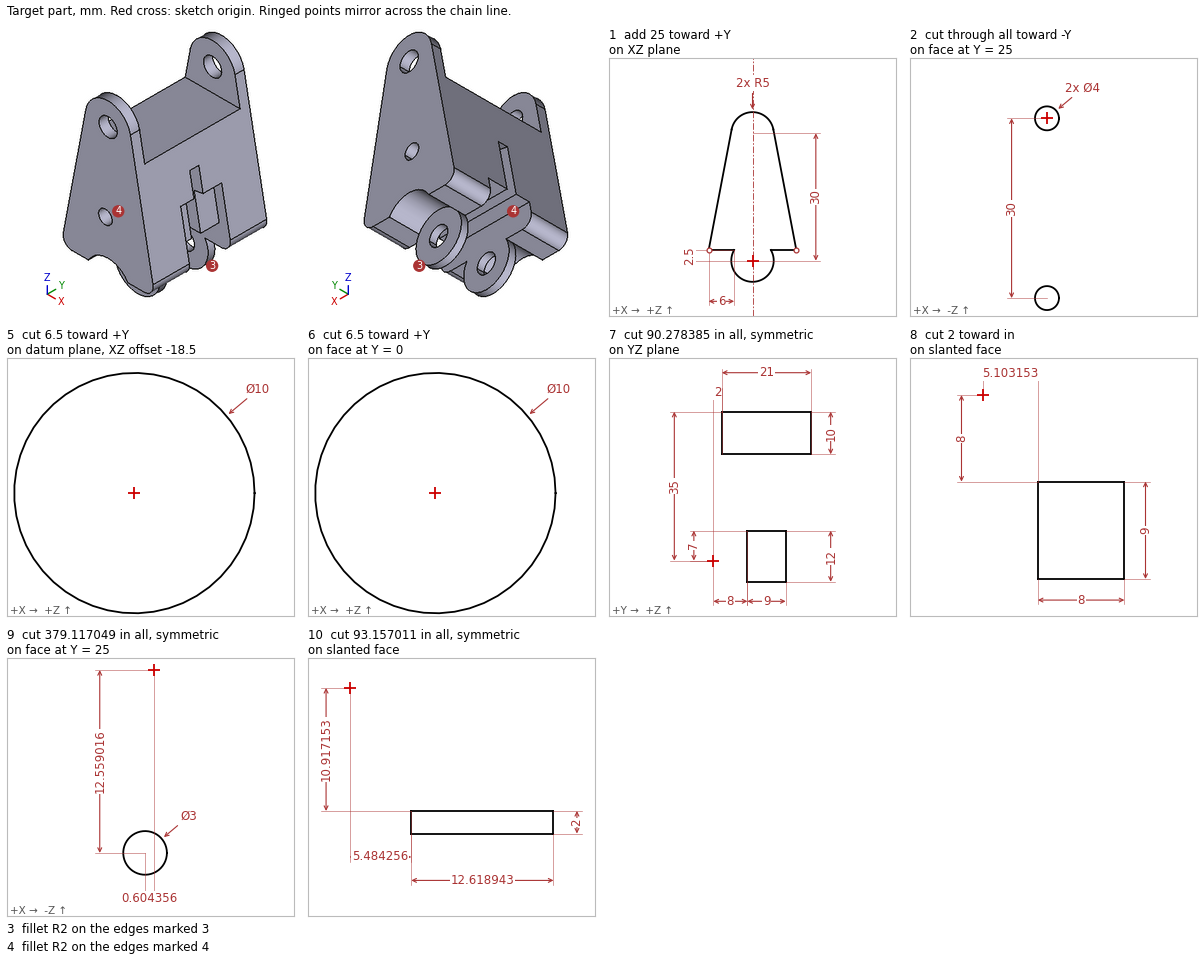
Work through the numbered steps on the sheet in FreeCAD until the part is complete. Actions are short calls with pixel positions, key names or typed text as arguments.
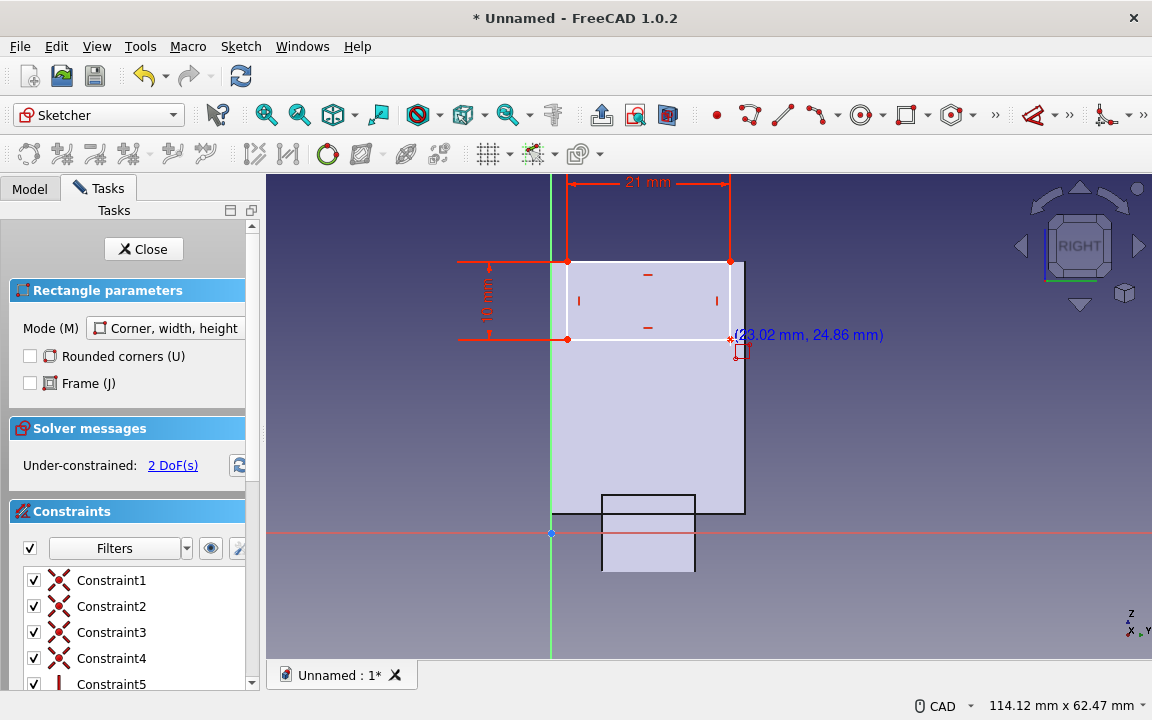
click(613, 479)
move(683, 572)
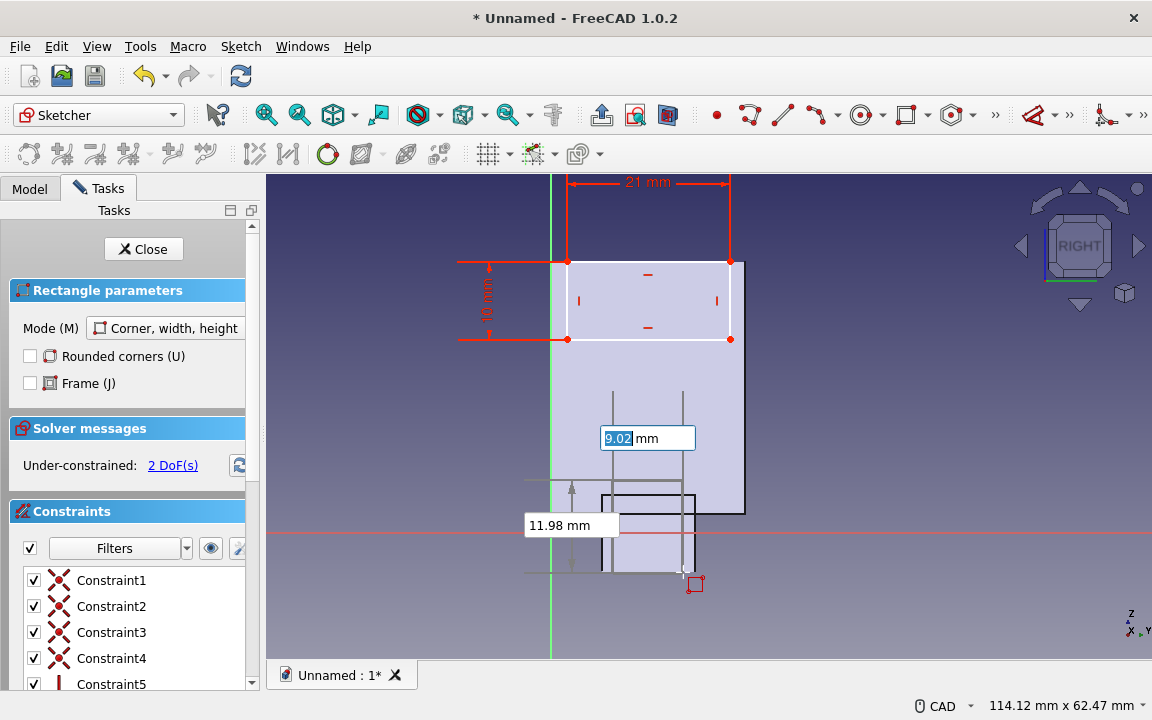
text(9)
key(Tab)
text(12)
key(Return)
key(Escape)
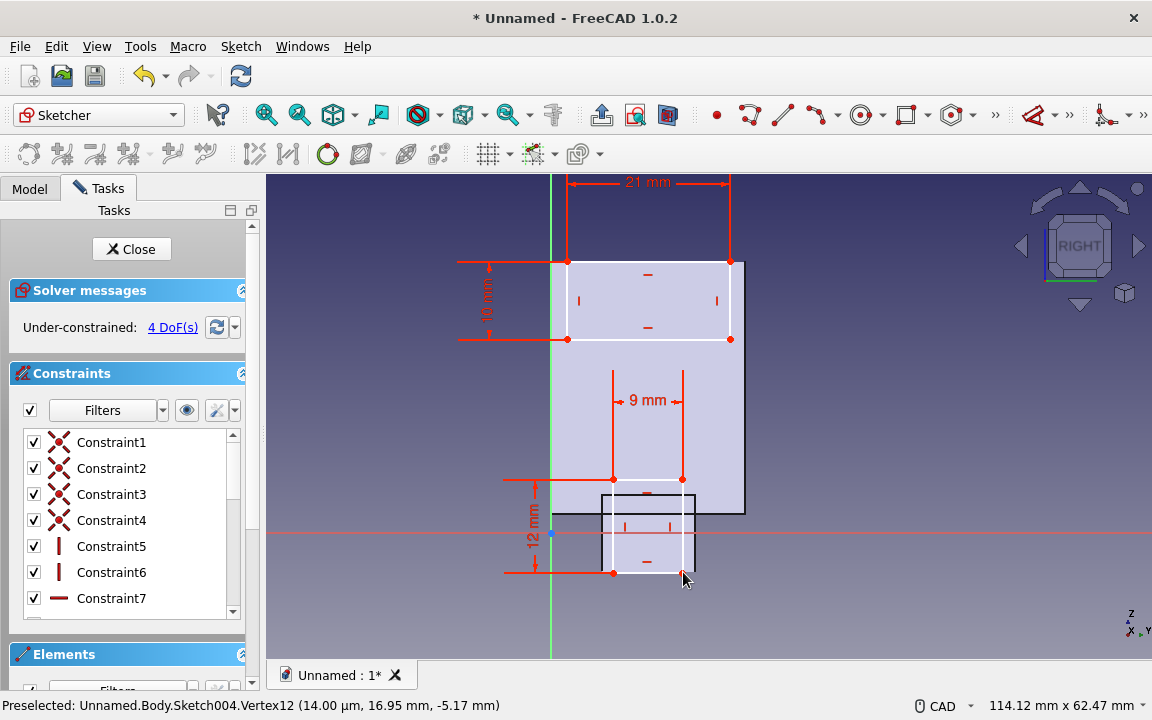
key(d)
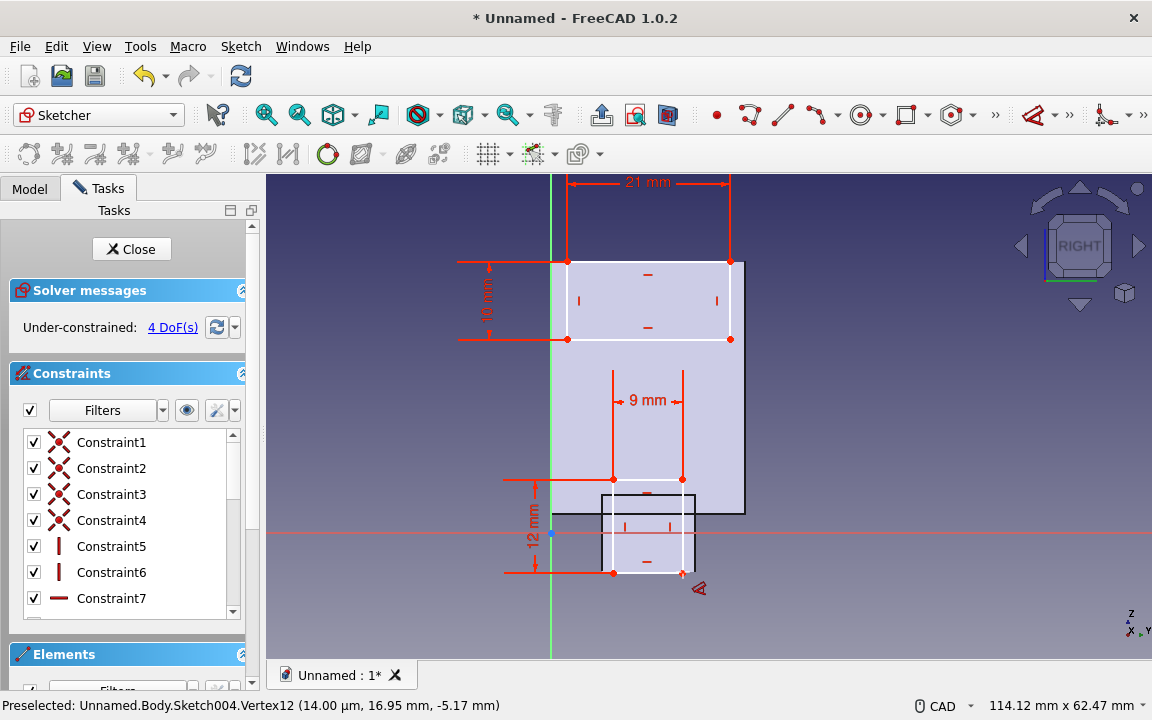
scroll(567, 262, up, 5)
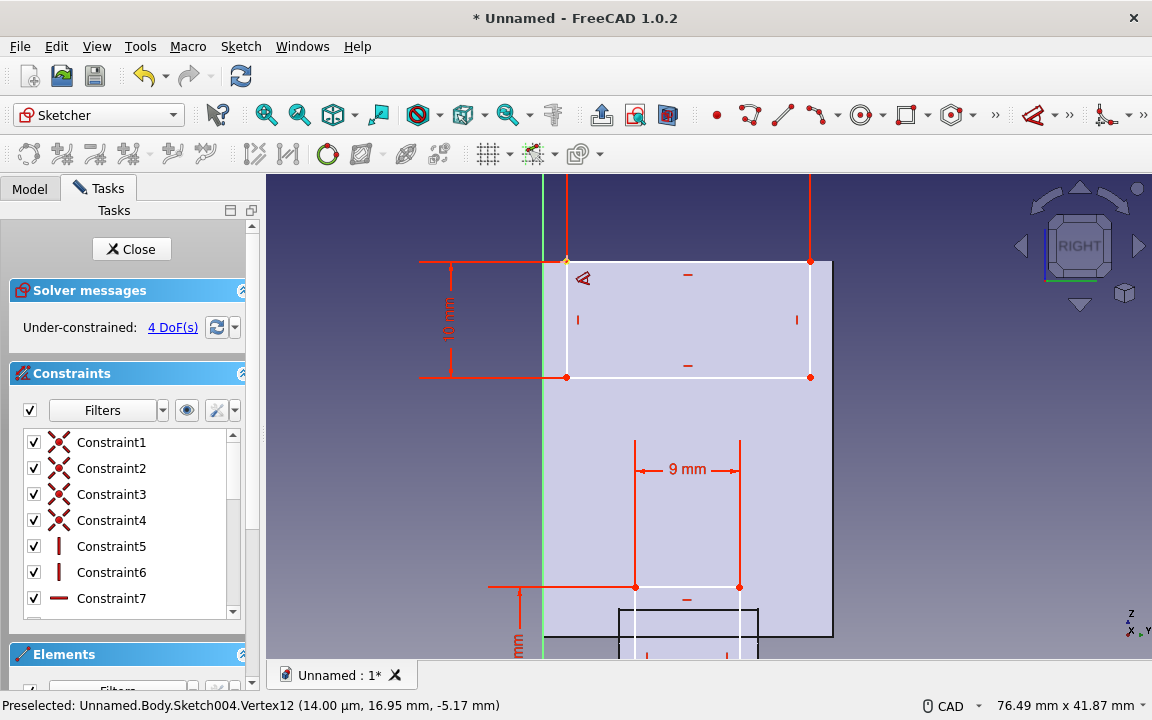
click(566, 262)
click(545, 228)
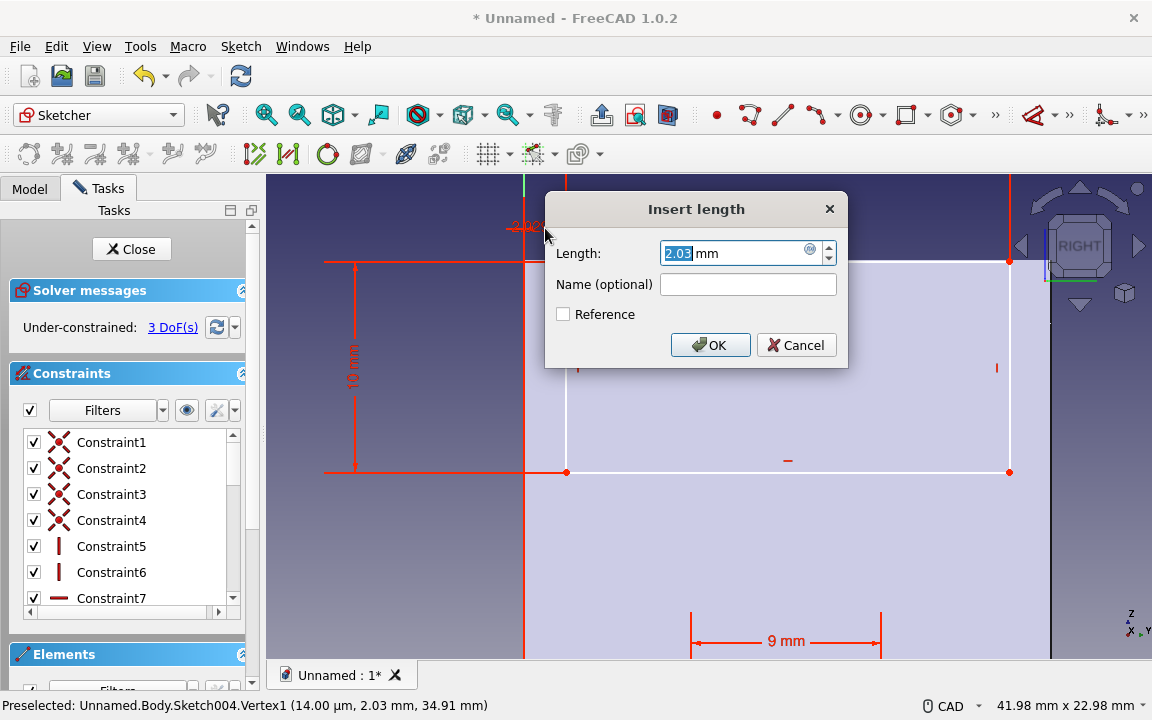
text(2)
key(Return)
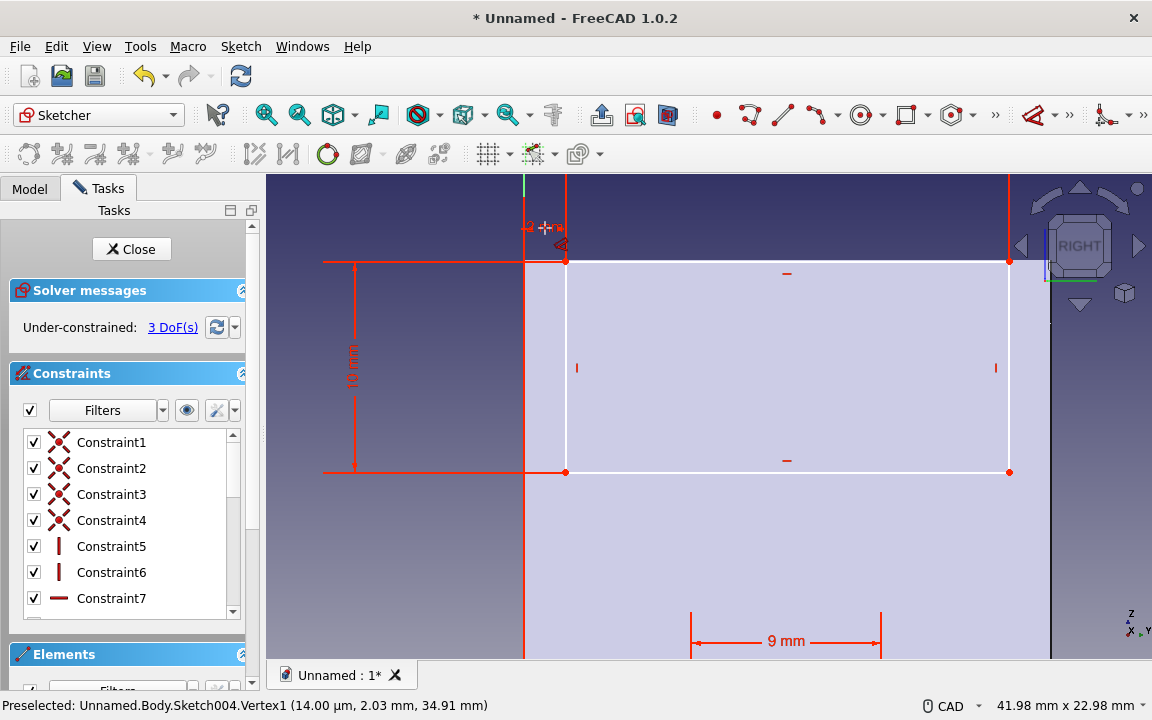
scroll(567, 262, down, 5)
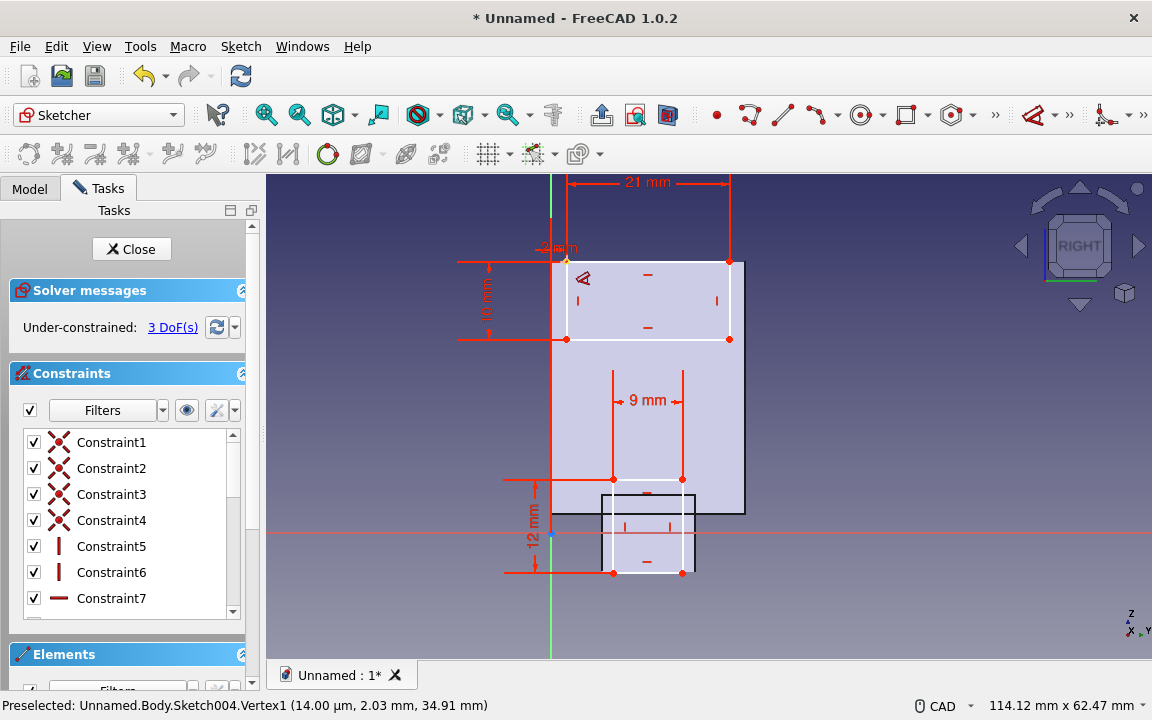
click(613, 480)
click(582, 567)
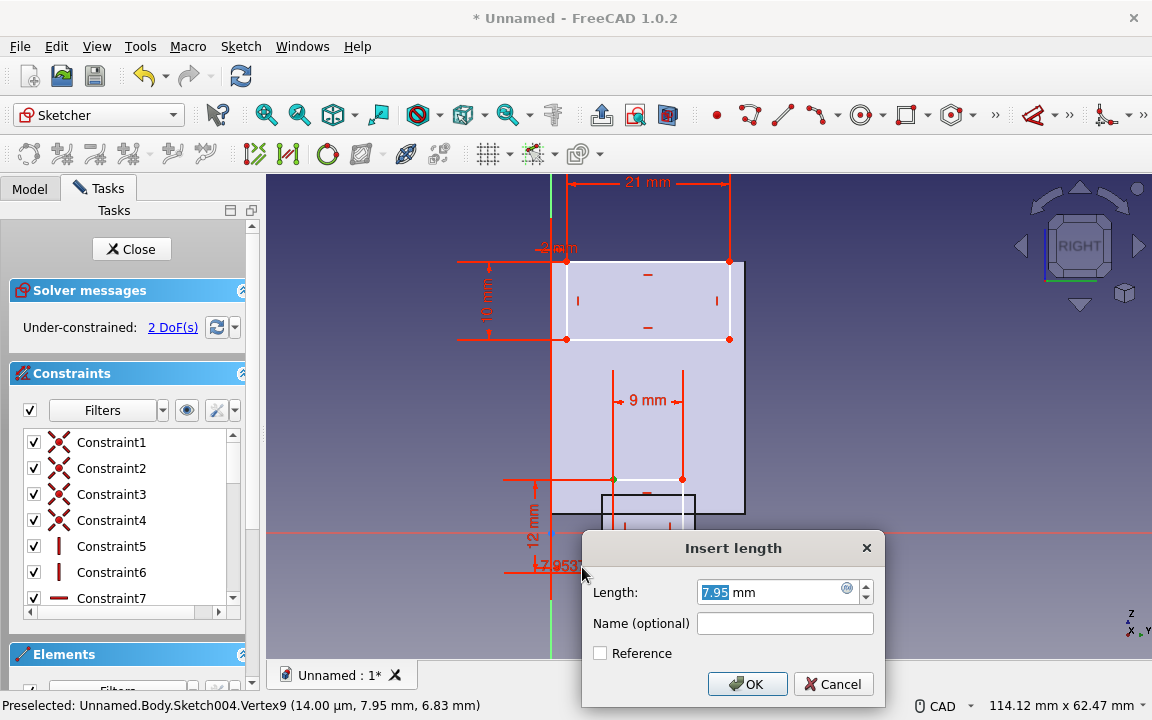
text(8)
key(Return)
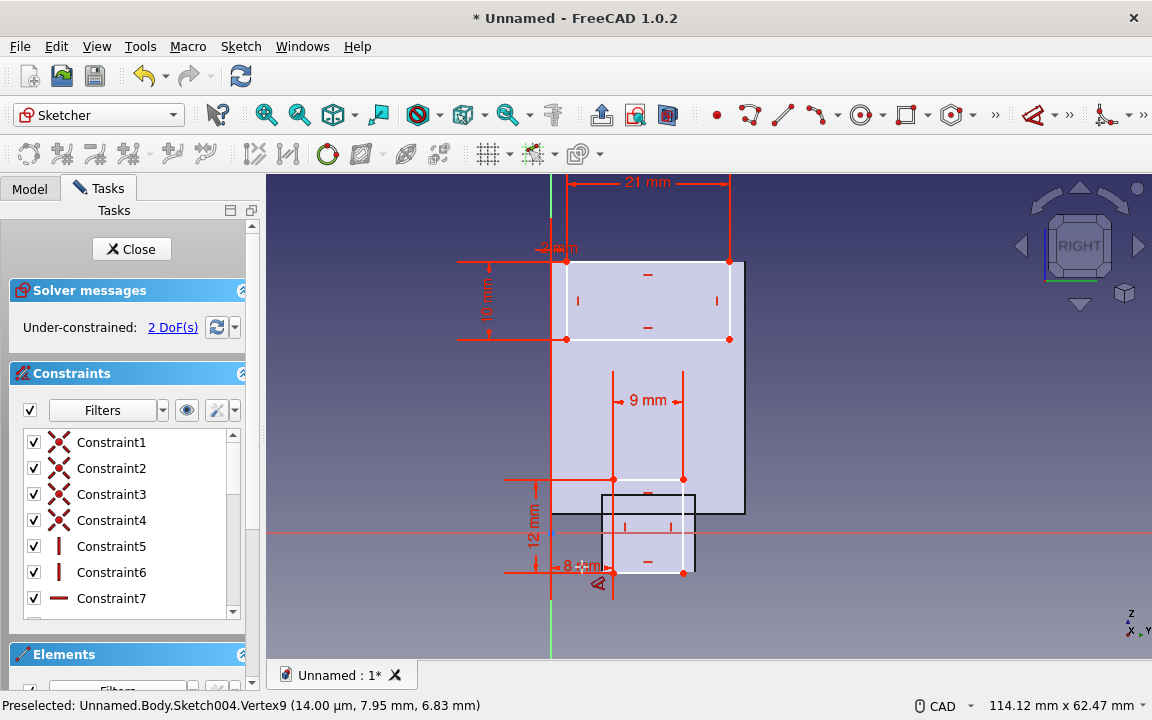
click(613, 480)
click(517, 507)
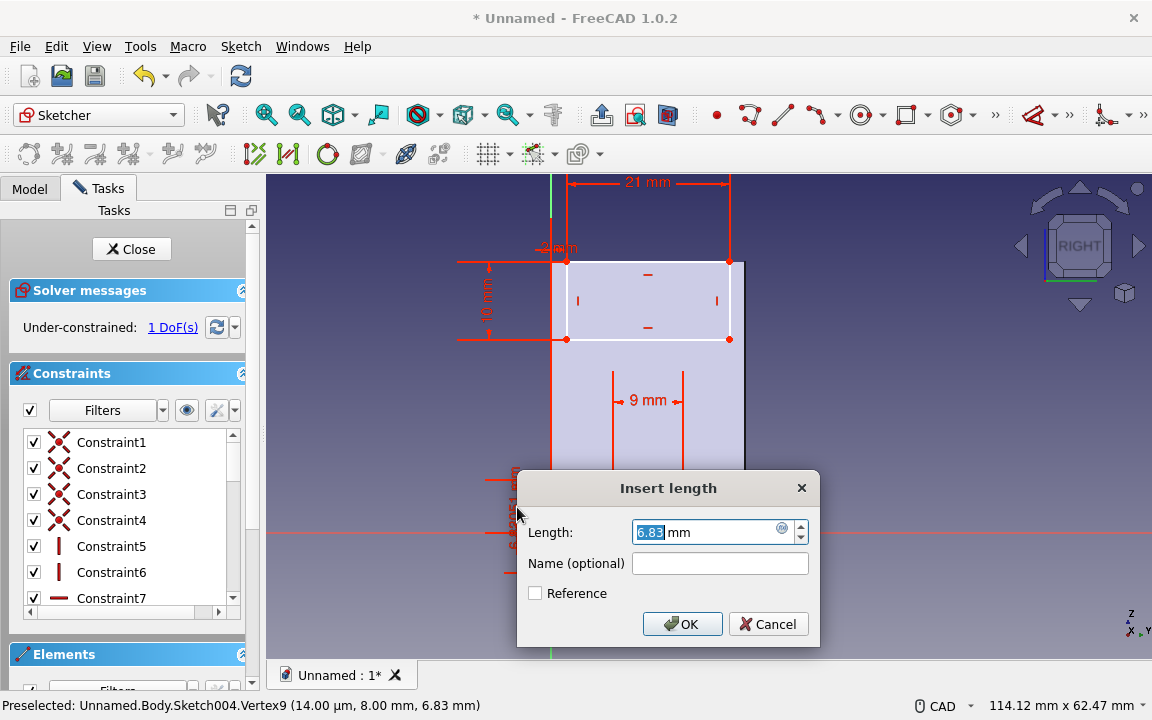
text(7)
key(Return)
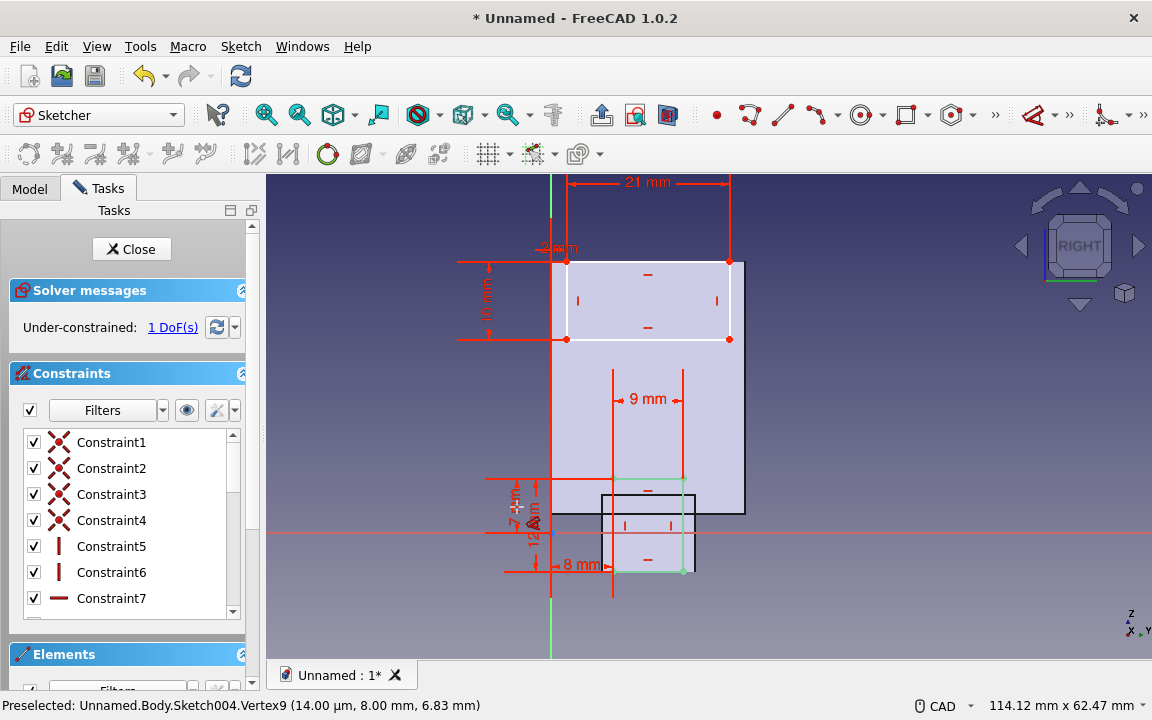
click(567, 262)
click(517, 398)